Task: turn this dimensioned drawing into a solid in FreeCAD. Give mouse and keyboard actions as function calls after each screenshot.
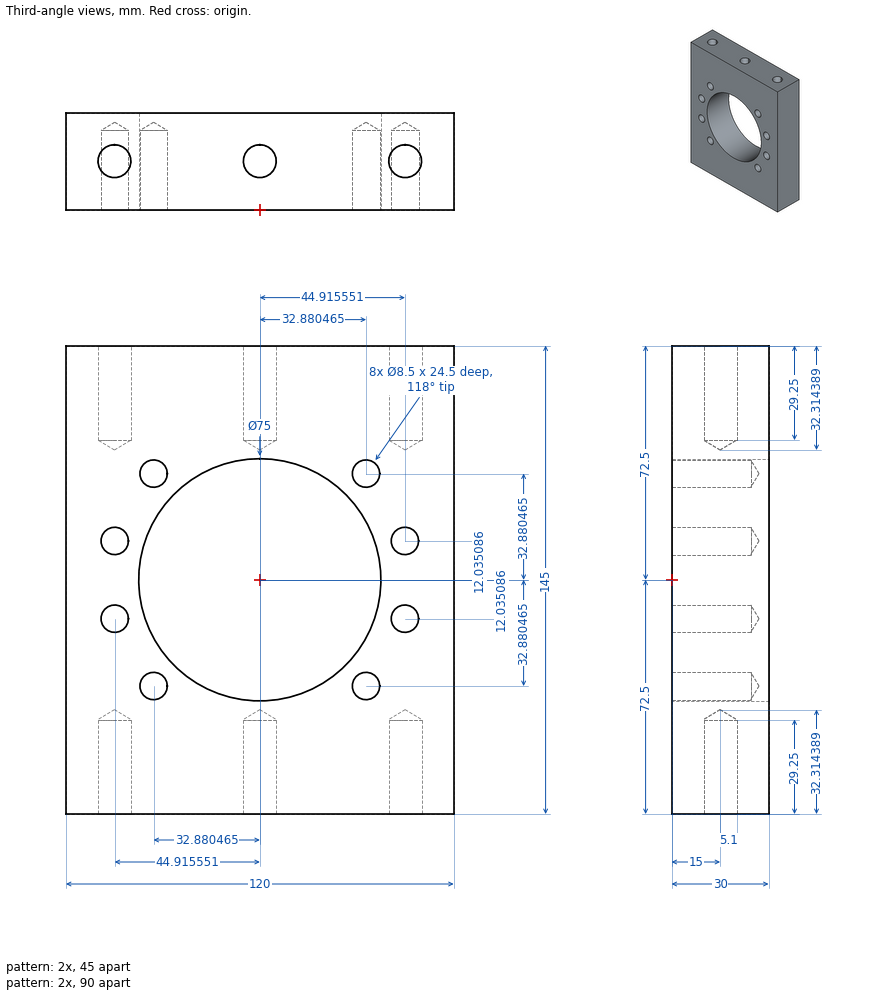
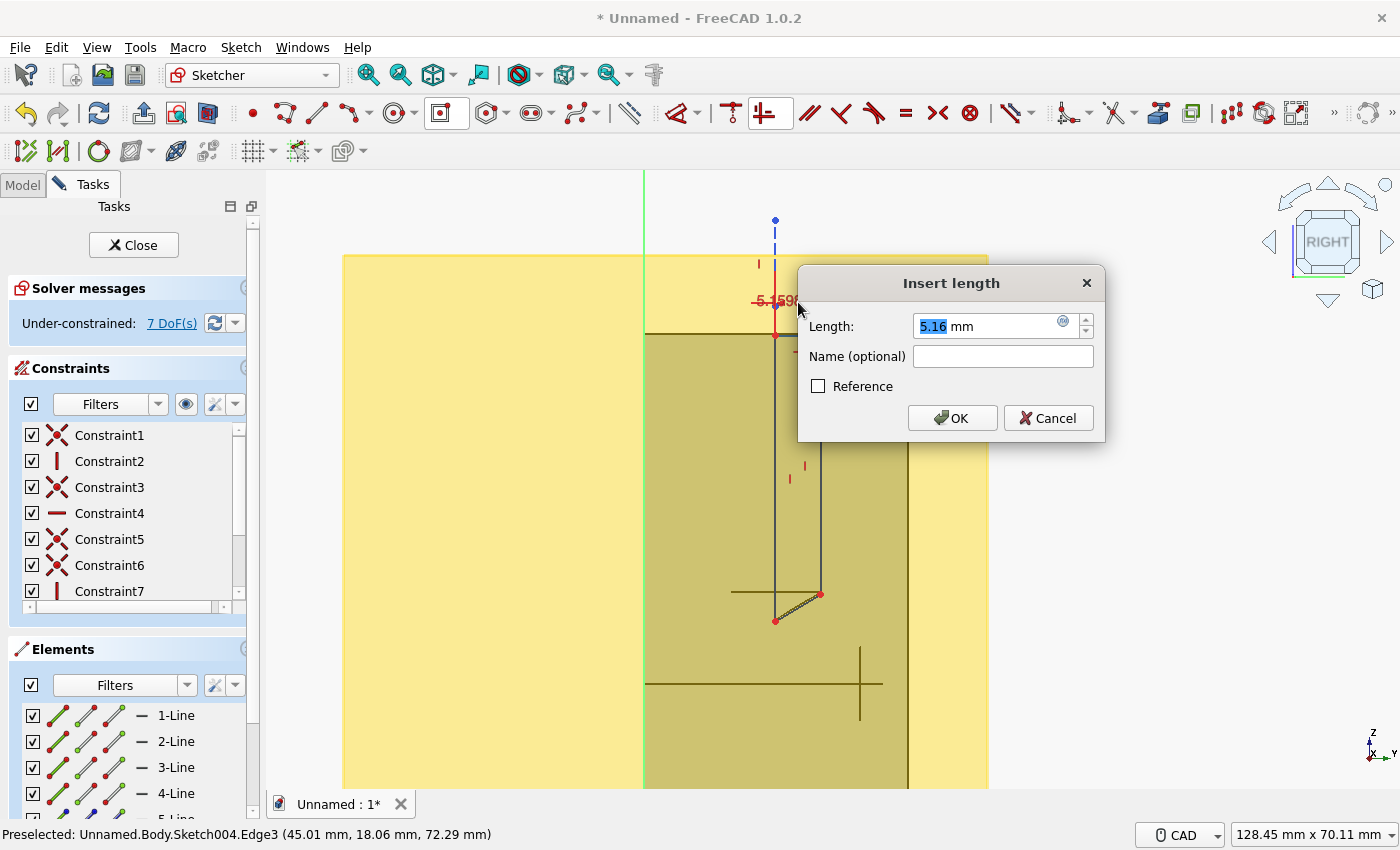
text(5.1)
key(Return)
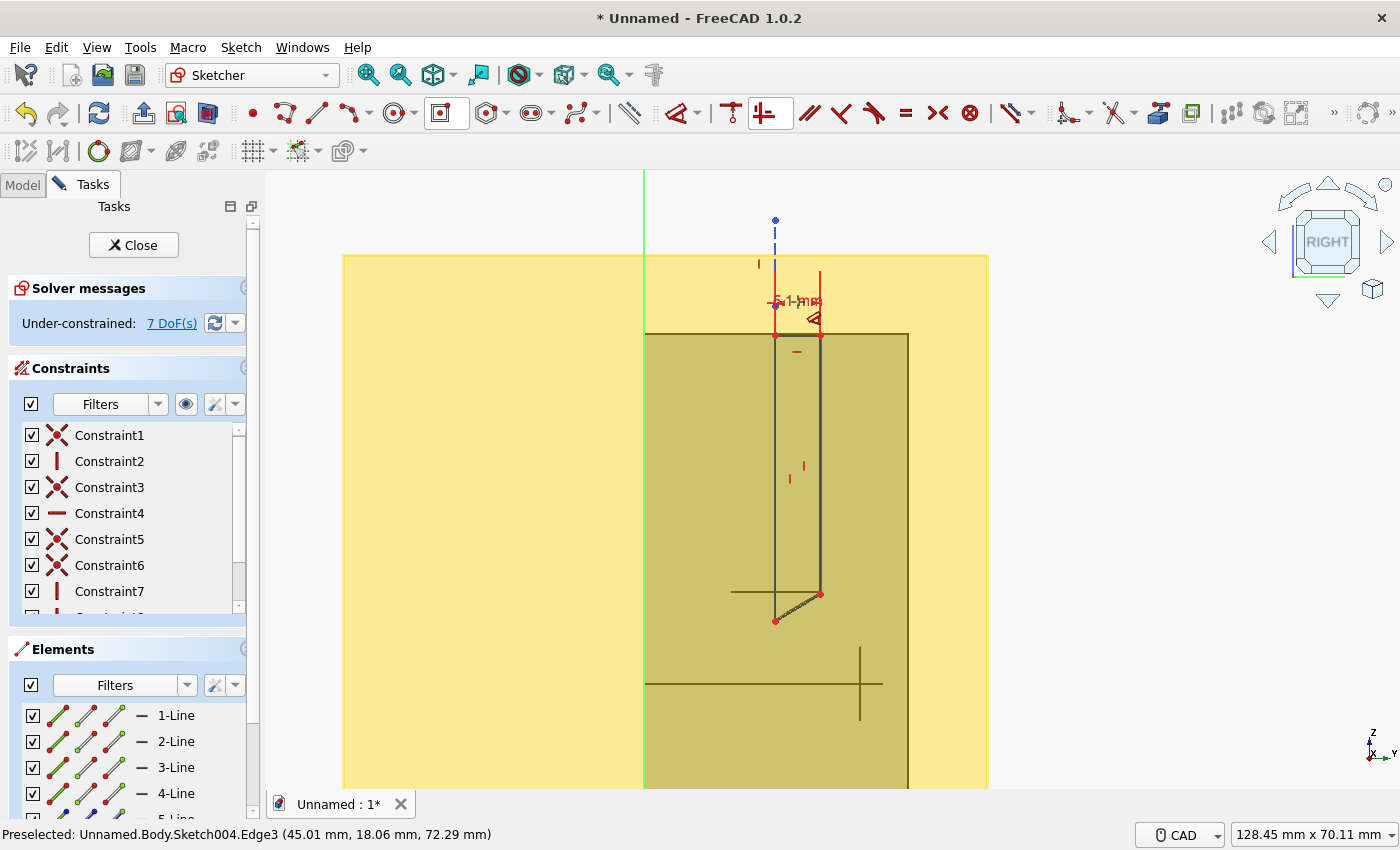
click(775, 622)
click(709, 588)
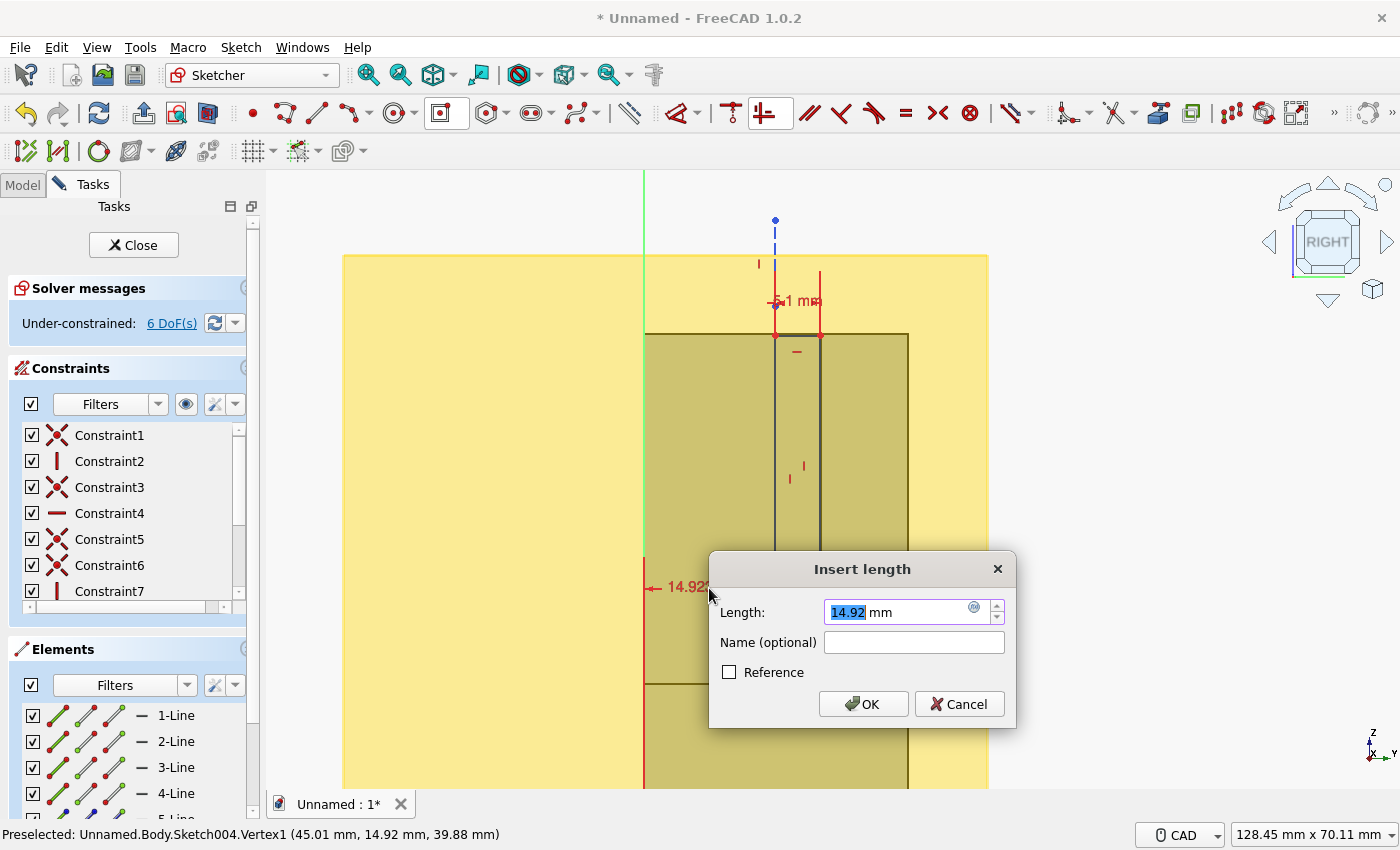
text(15)
key(Return)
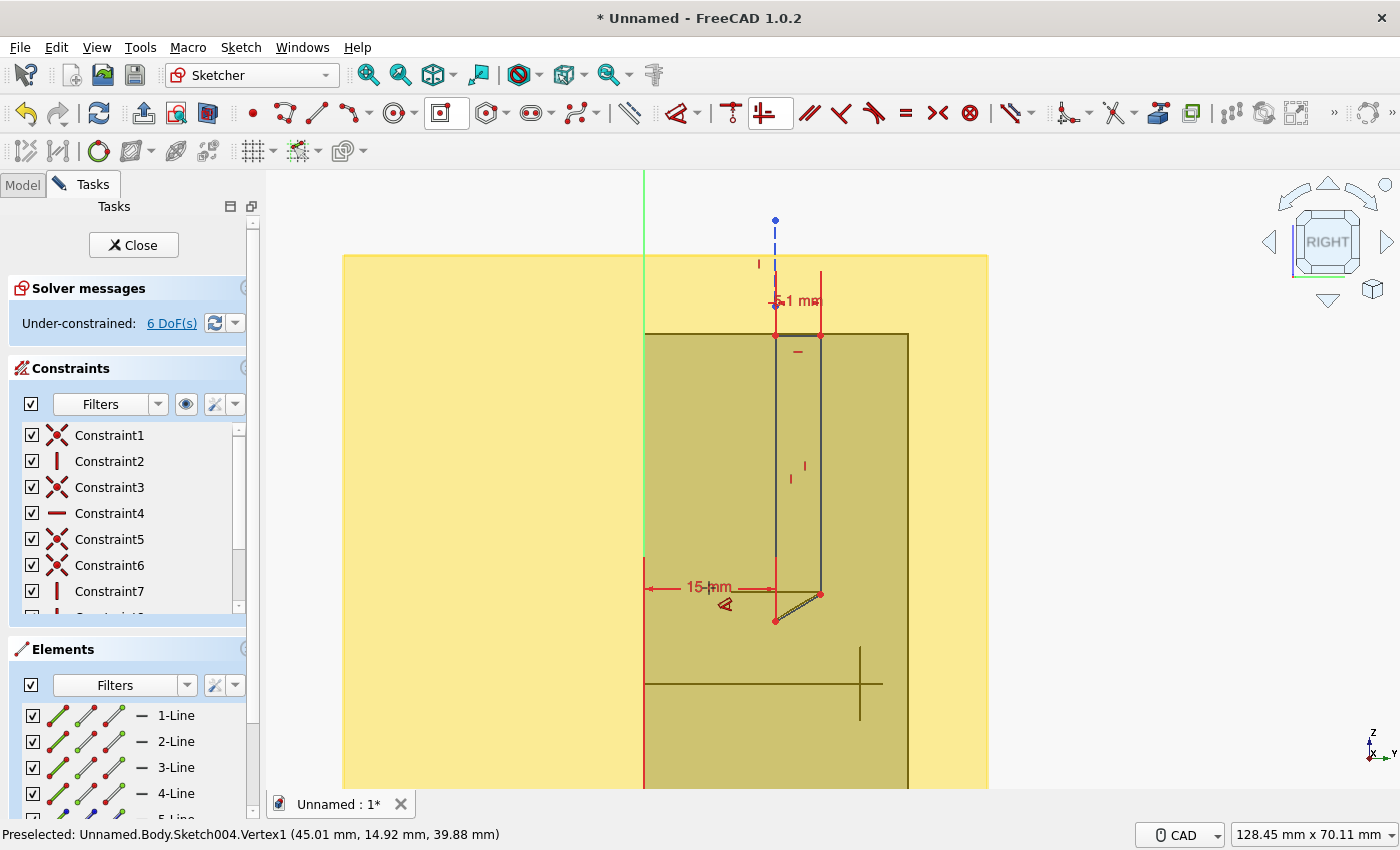
click(775, 307)
click(709, 273)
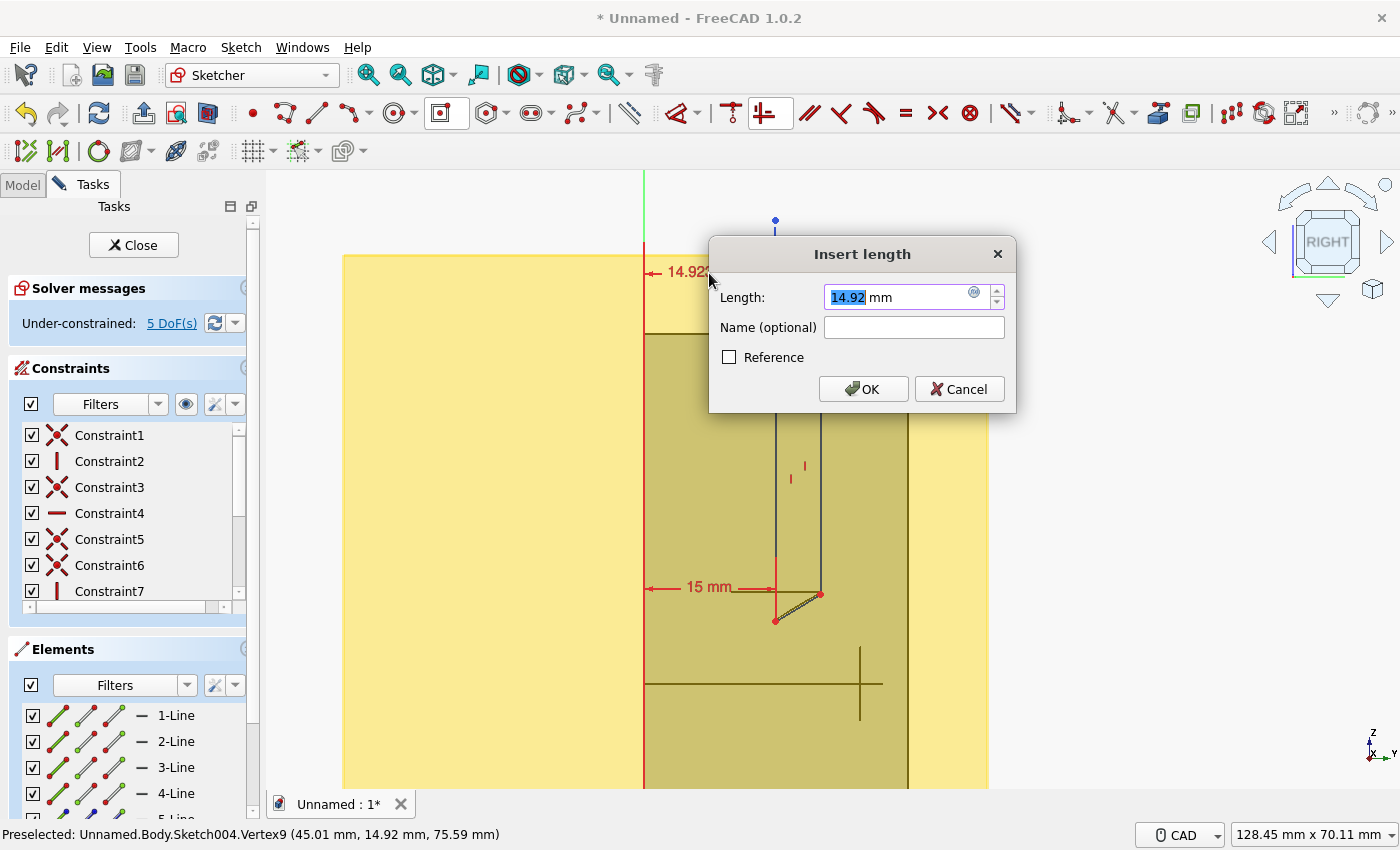
text(15)
key(Return)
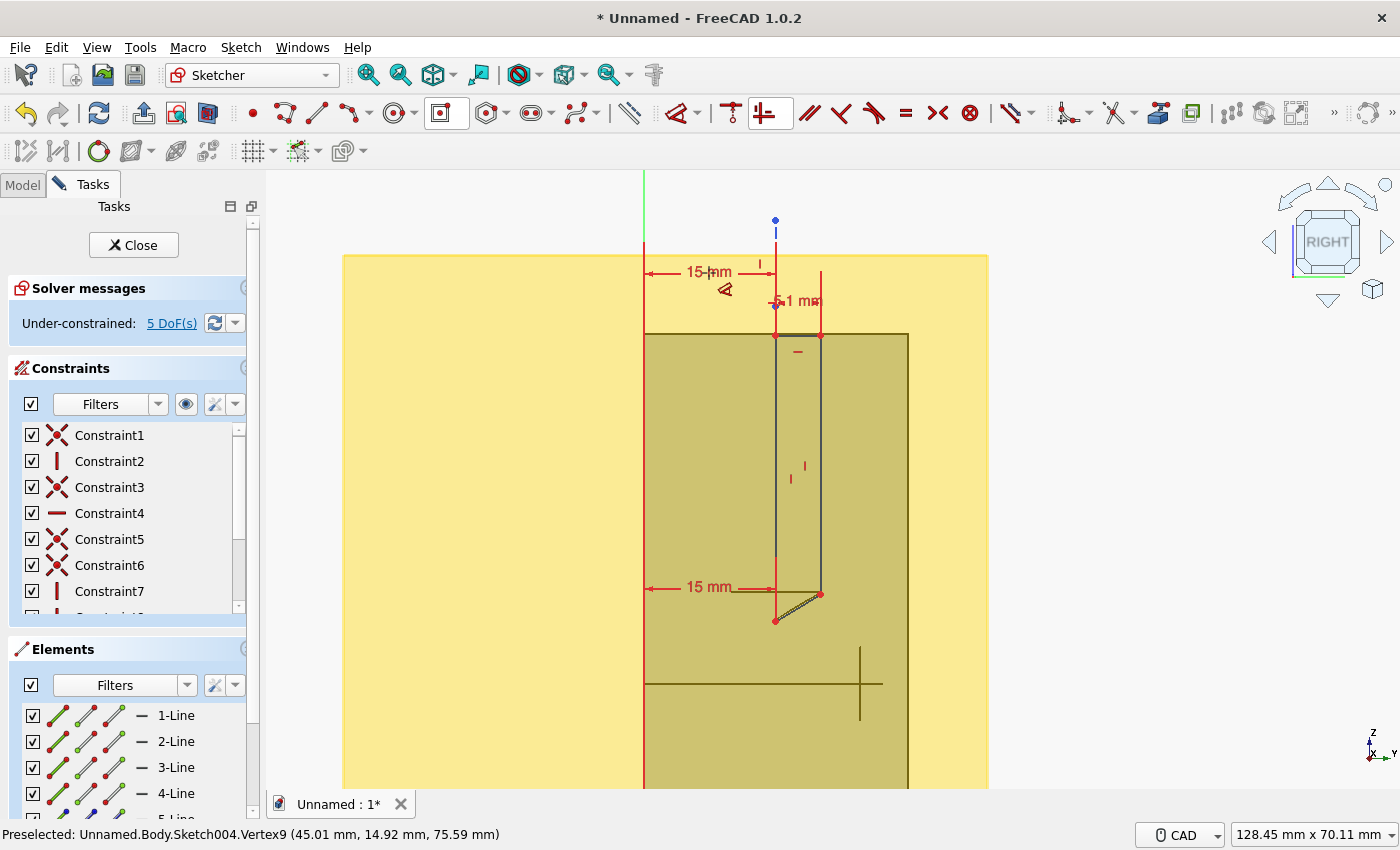
click(821, 517)
click(855, 465)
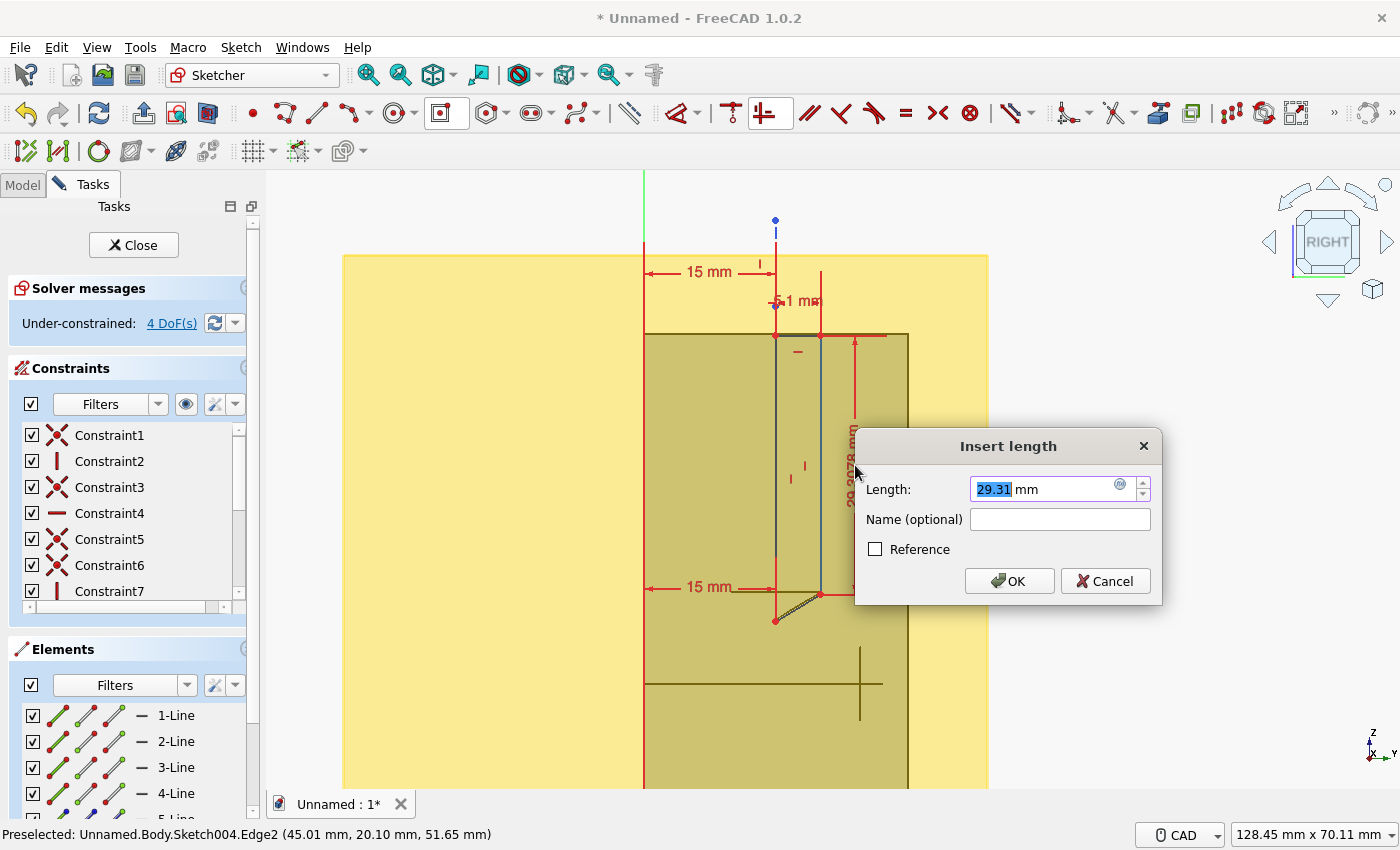
text(29.25)
key(Return)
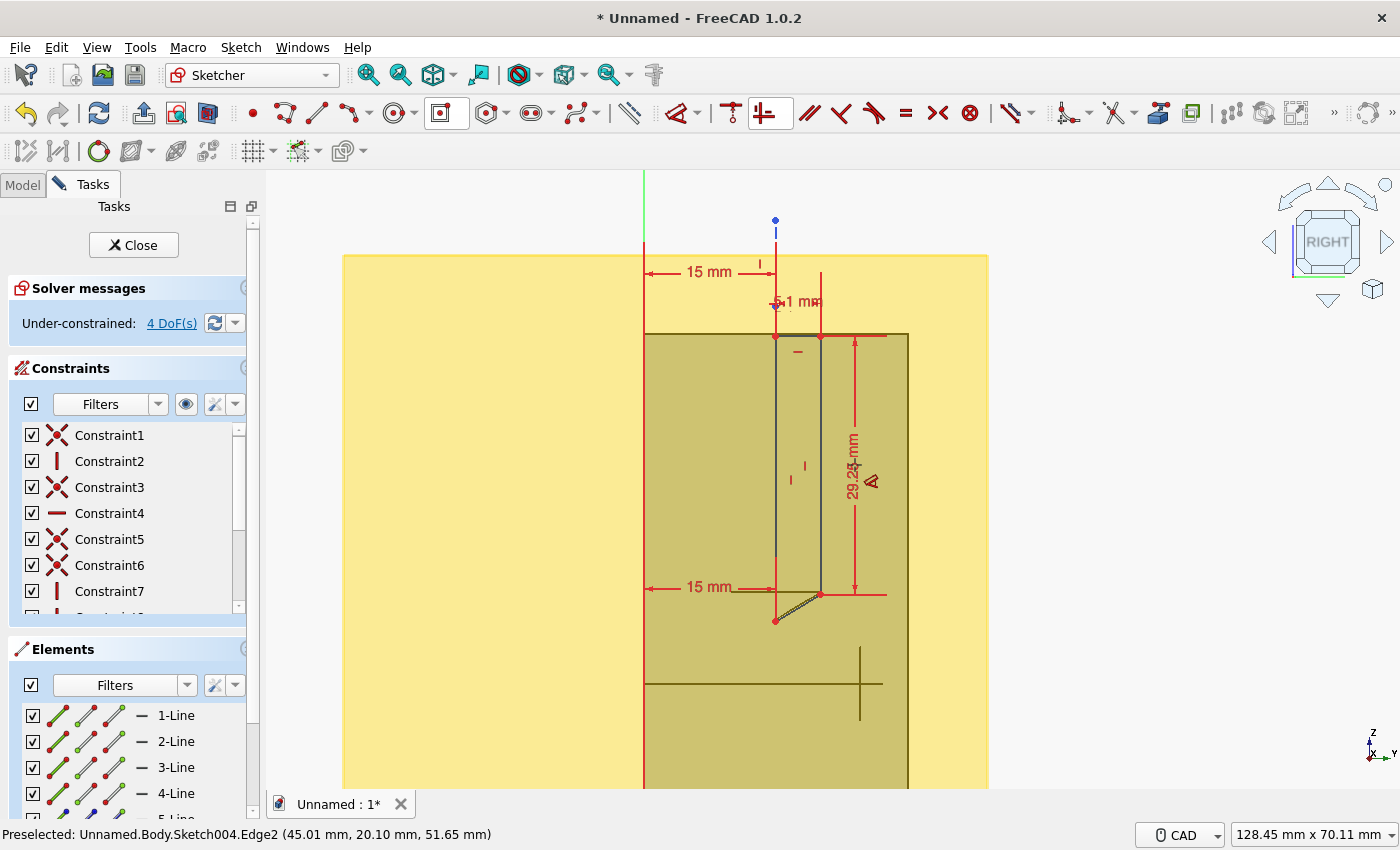
click(821, 336)
click(855, 549)